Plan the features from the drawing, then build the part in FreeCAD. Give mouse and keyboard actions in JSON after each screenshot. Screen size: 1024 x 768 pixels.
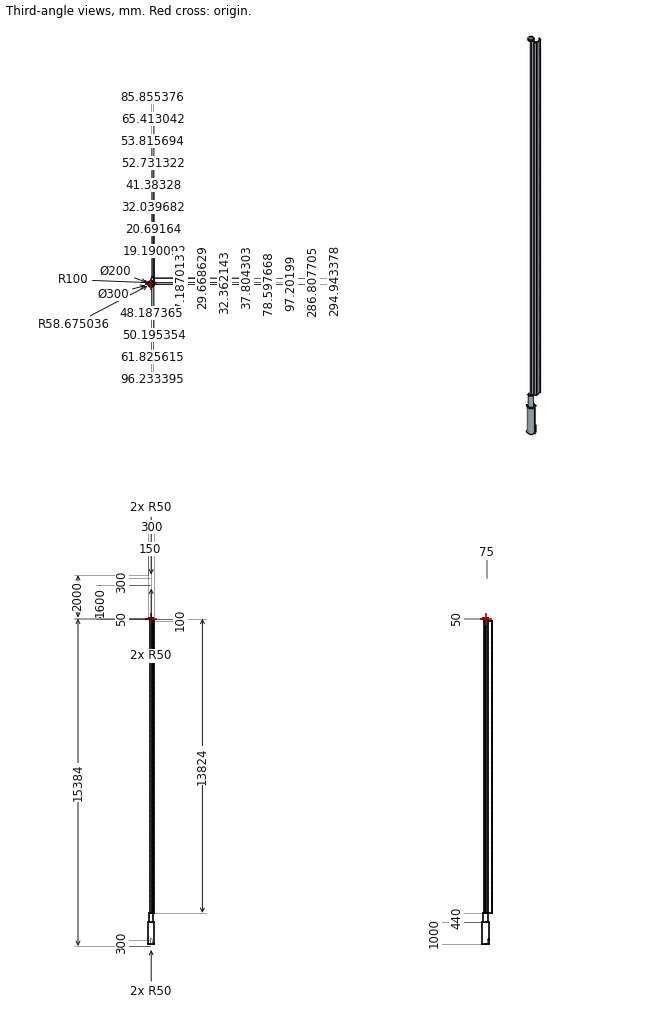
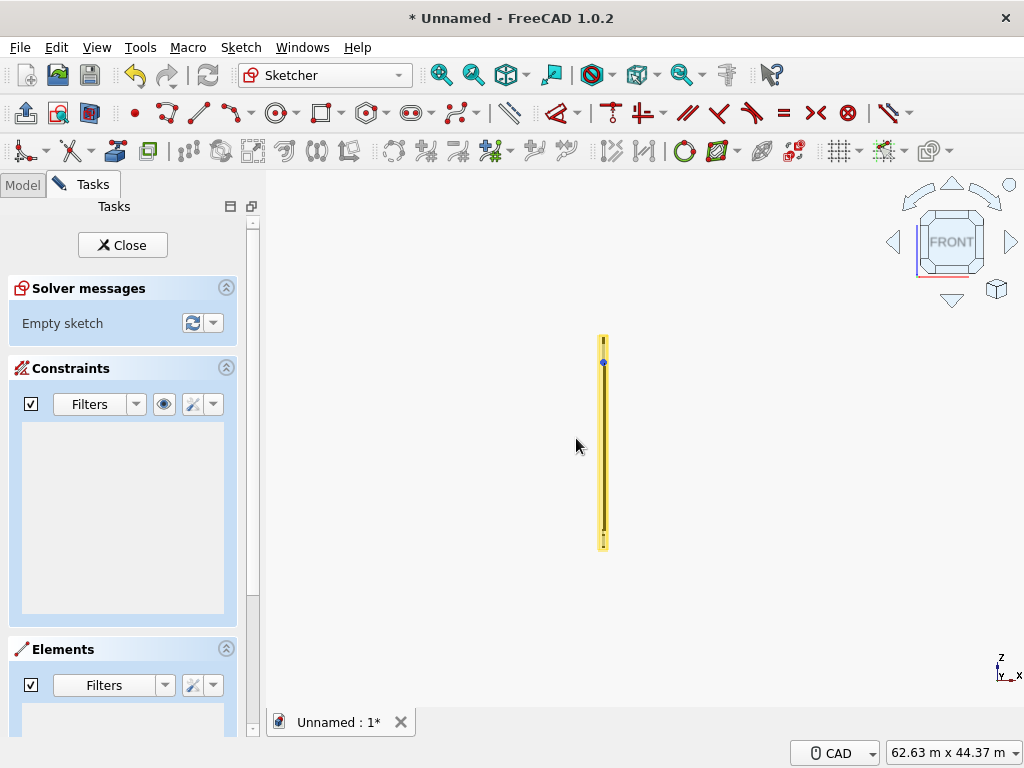
{"action": "scroll", "coordinate": [605, 553], "scroll_direction": "up", "scroll_amount": 15}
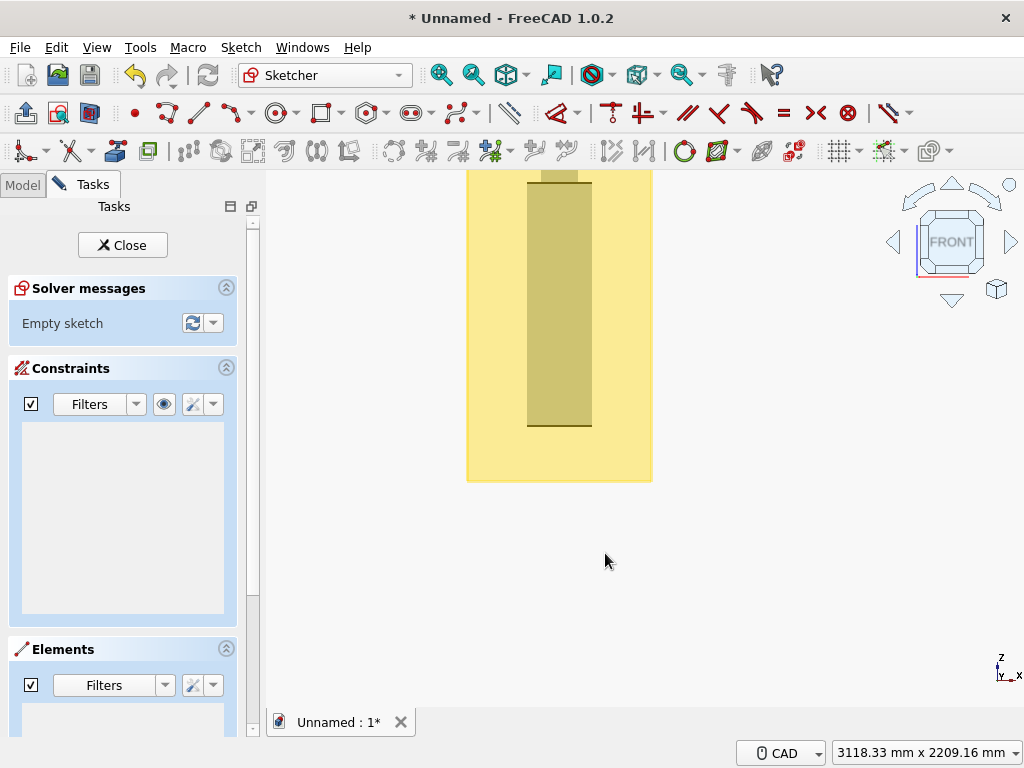
{"action": "scroll", "coordinate": [552, 410], "scroll_direction": "up", "scroll_amount": 6}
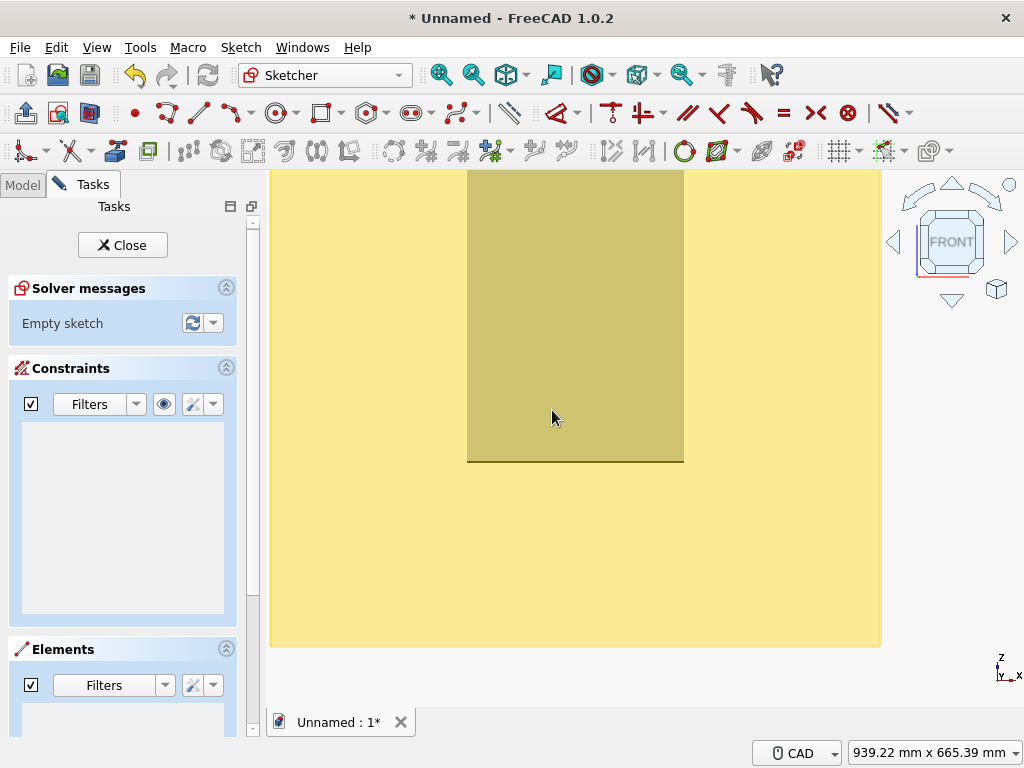
{"action": "left_click", "coordinate": [412, 114]}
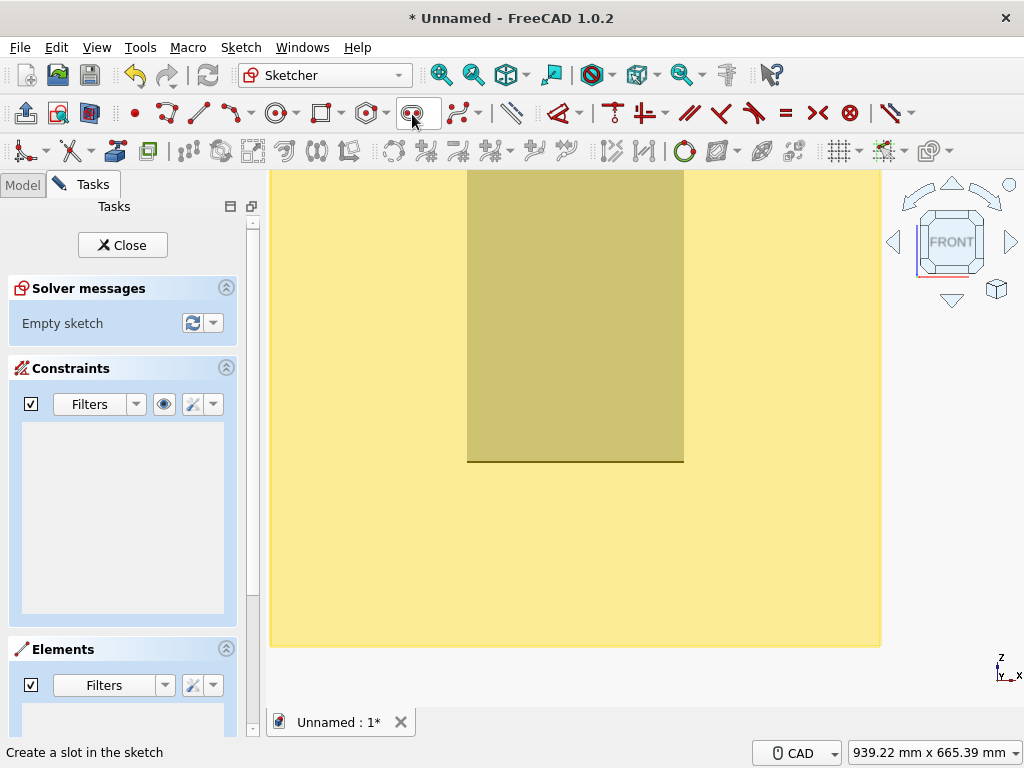
{"action": "left_click", "coordinate": [575, 559]}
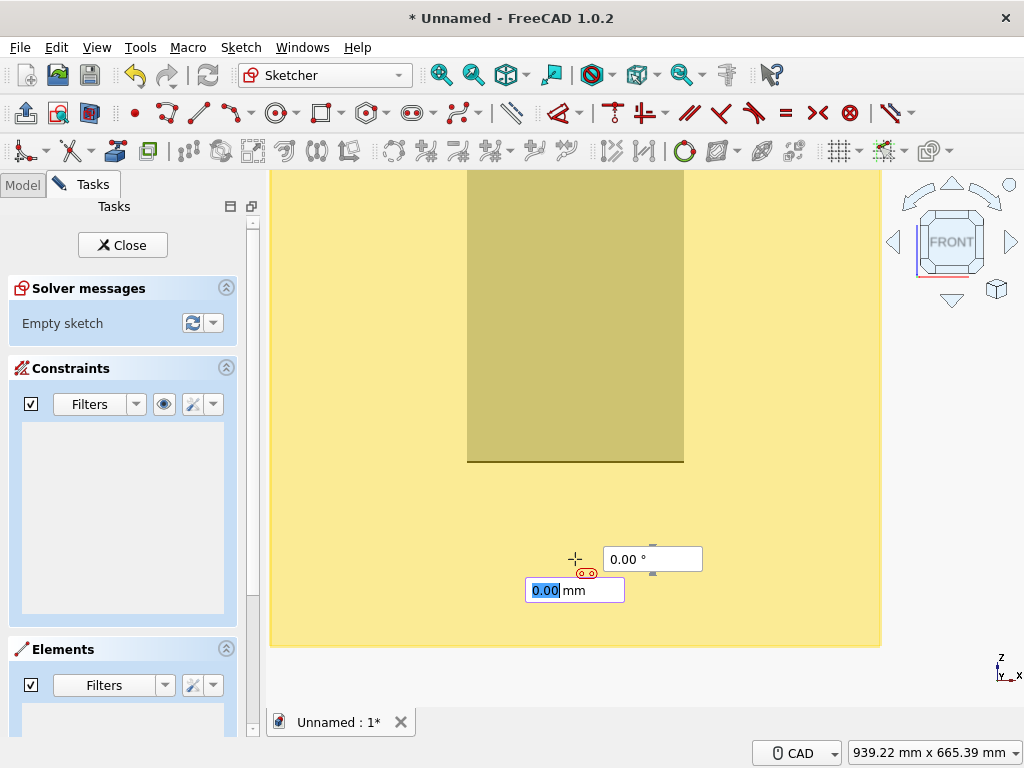
{"action": "left_click", "coordinate": [584, 317]}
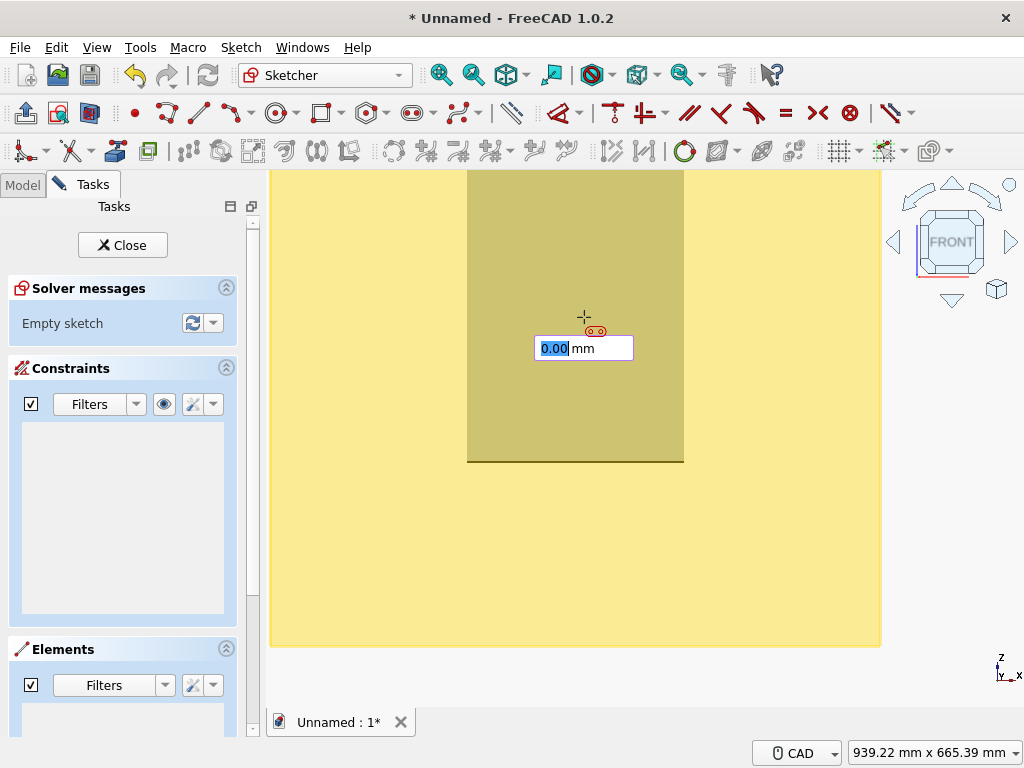
{"action": "left_click", "coordinate": [616, 438]}
{"action": "key", "text": "Escape"}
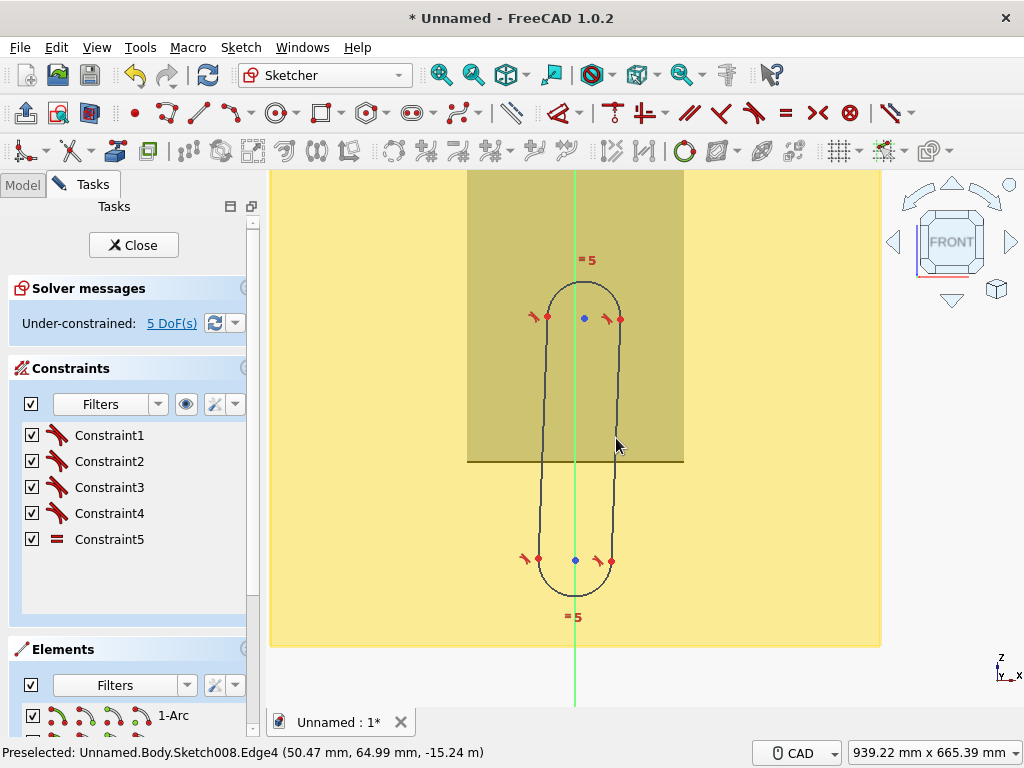
{"action": "left_click", "coordinate": [541, 486]}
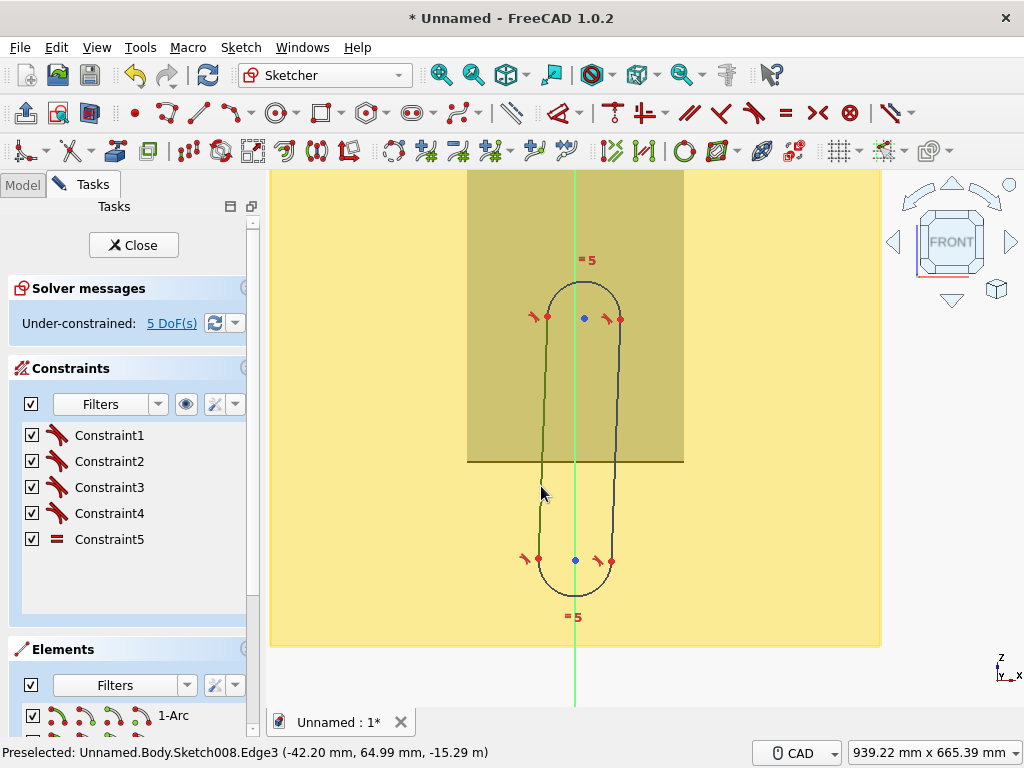
{"action": "key", "text": "v"}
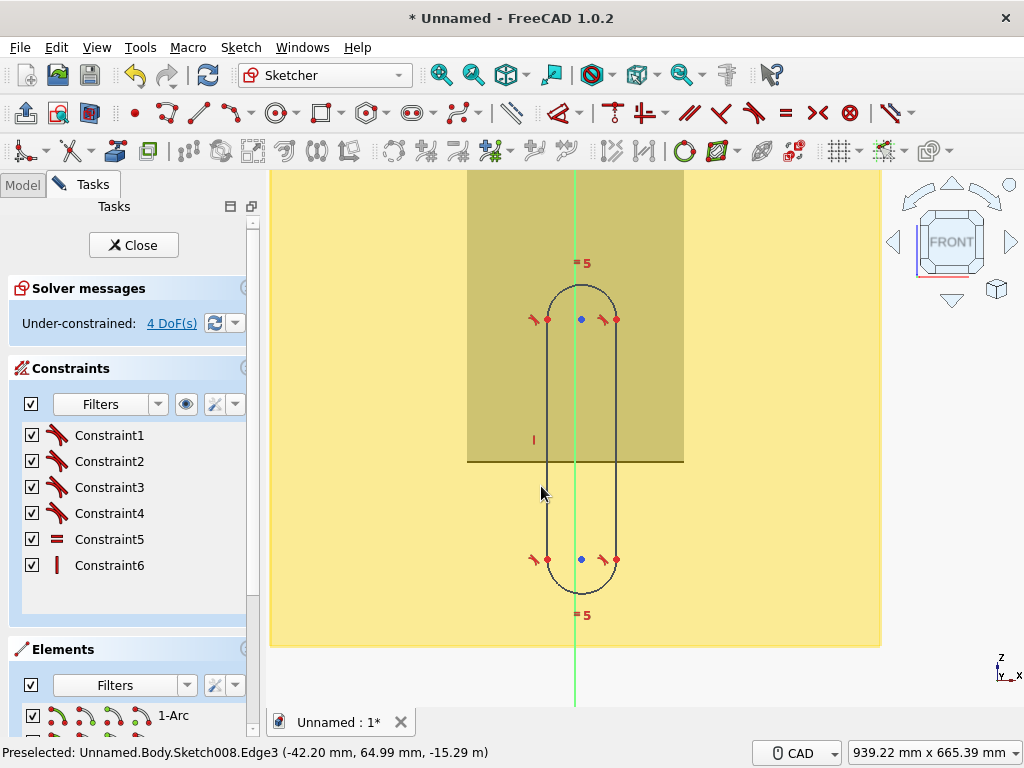
{"action": "left_click", "coordinate": [582, 559]}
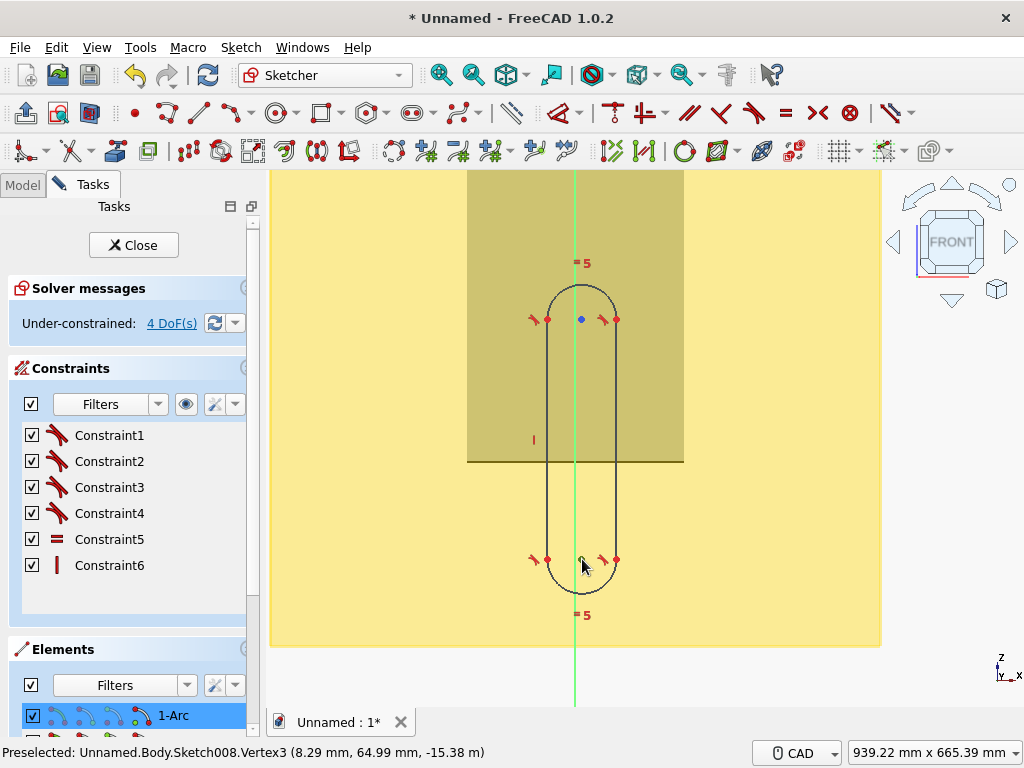
{"action": "left_click", "coordinate": [575, 645]}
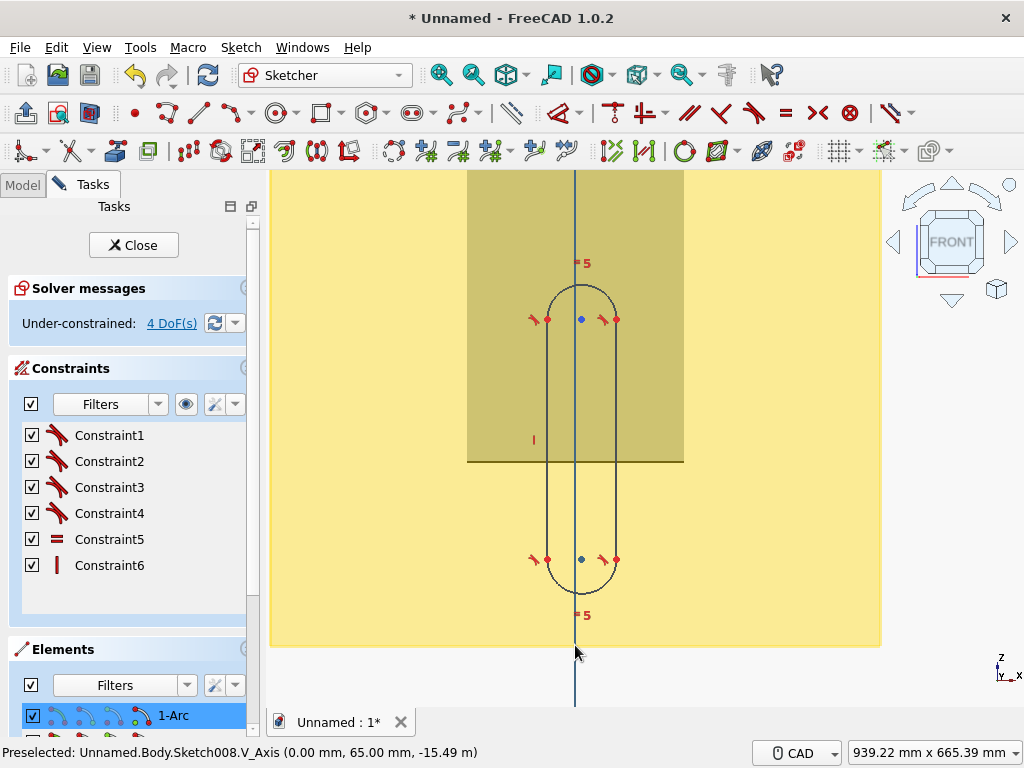
{"action": "left_click", "coordinate": [614, 114]}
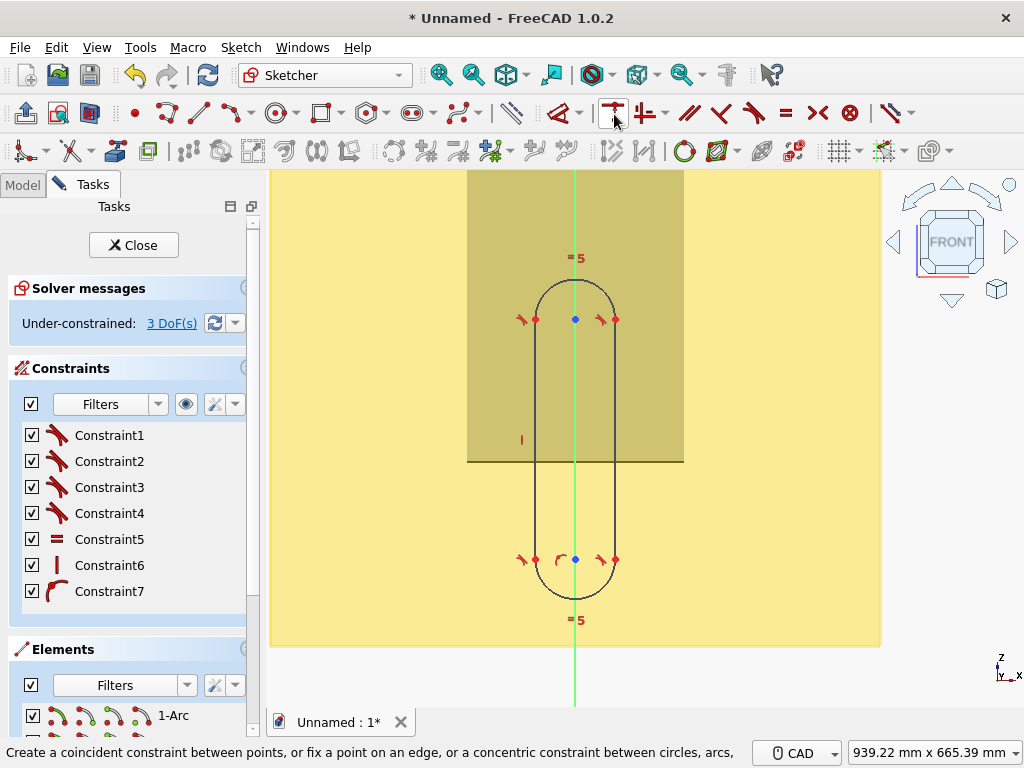
{"action": "left_click", "coordinate": [558, 114]}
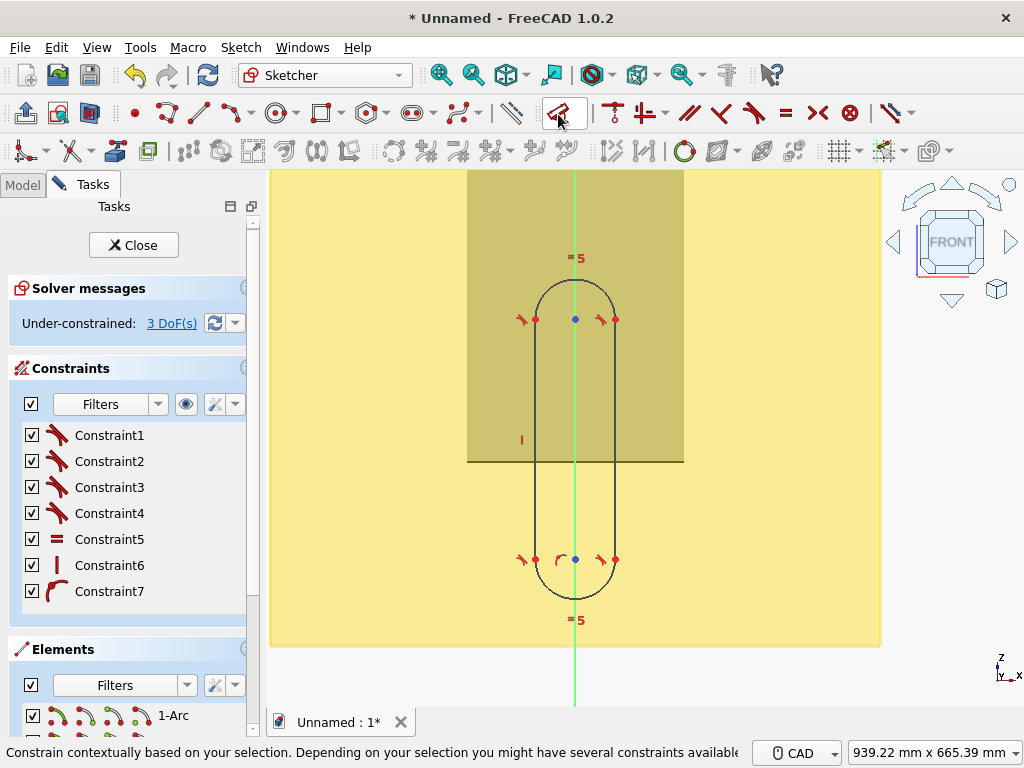
{"action": "left_click", "coordinate": [552, 591]}
{"action": "left_click", "coordinate": [533, 617]}